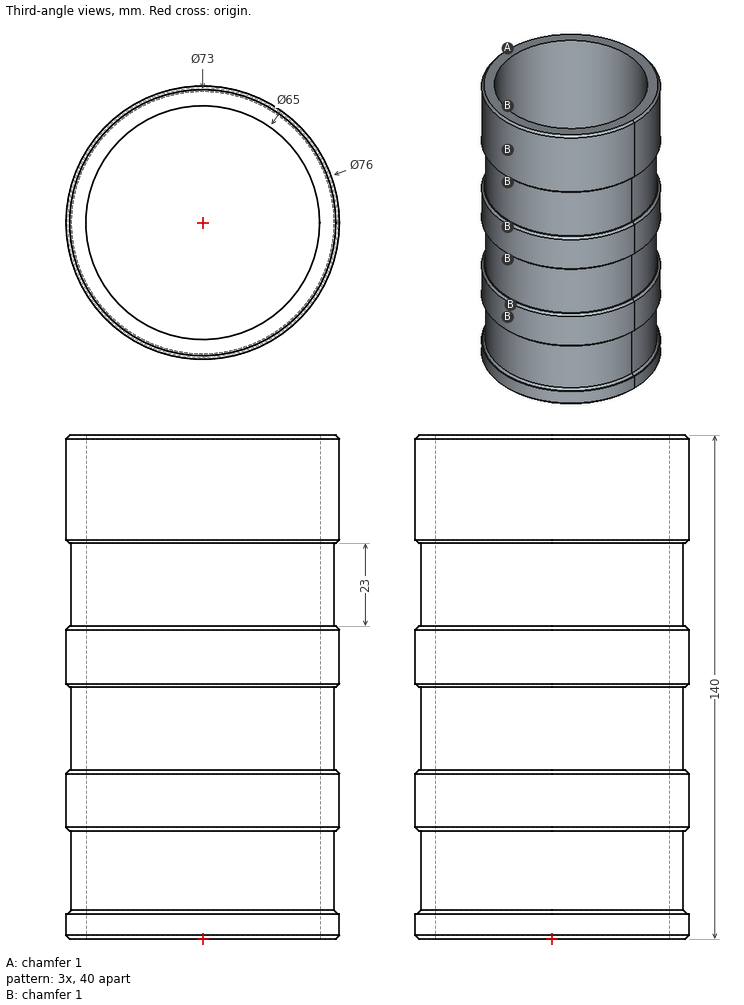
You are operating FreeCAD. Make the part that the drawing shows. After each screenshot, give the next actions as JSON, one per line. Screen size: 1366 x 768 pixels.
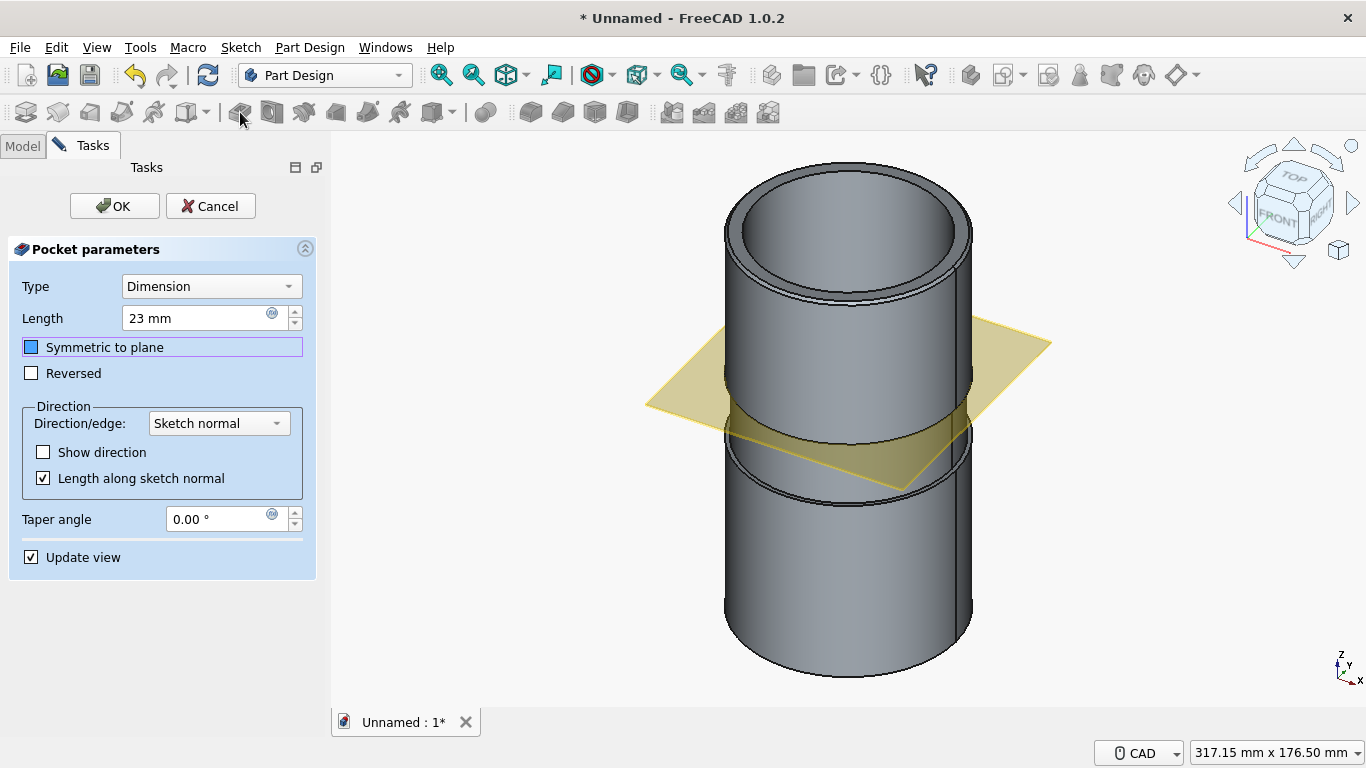
{"action": "left_click", "coordinate": [30, 373]}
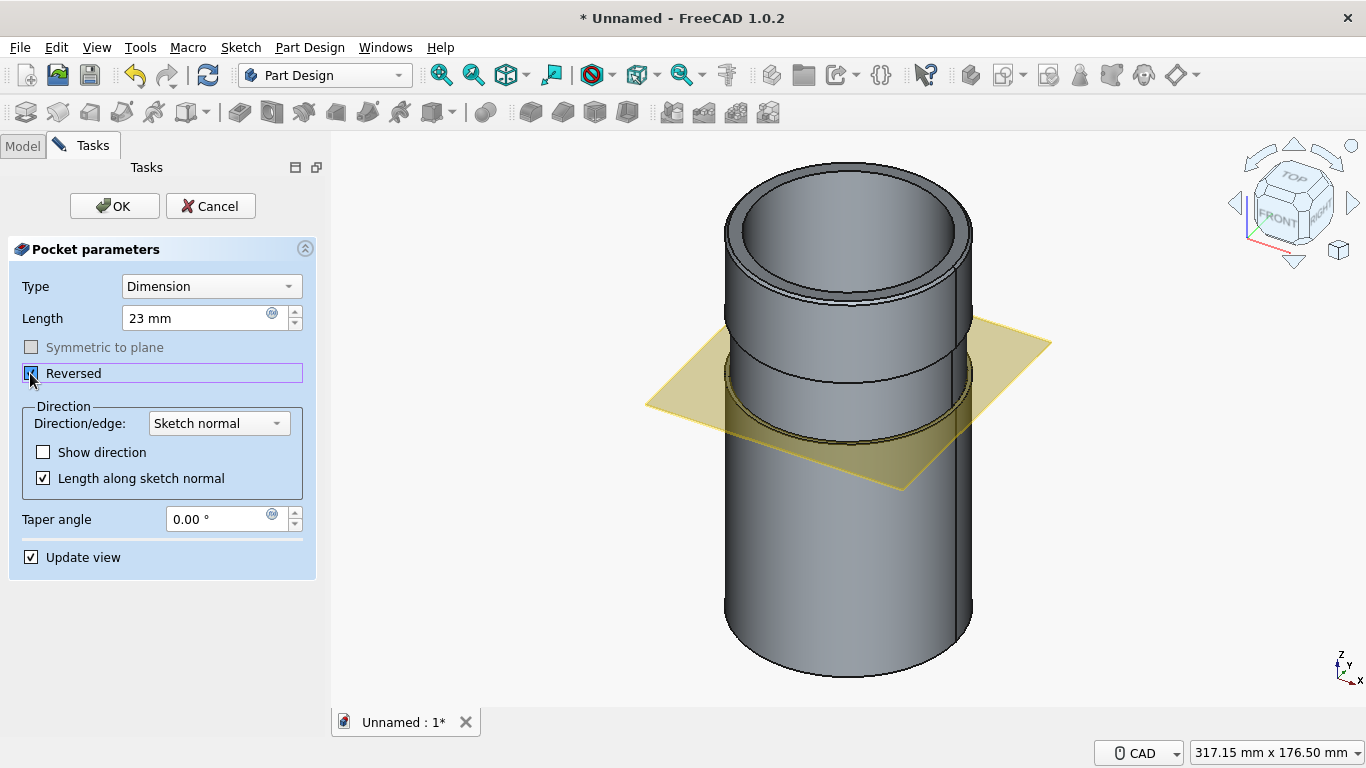
{"action": "left_click", "coordinate": [115, 206]}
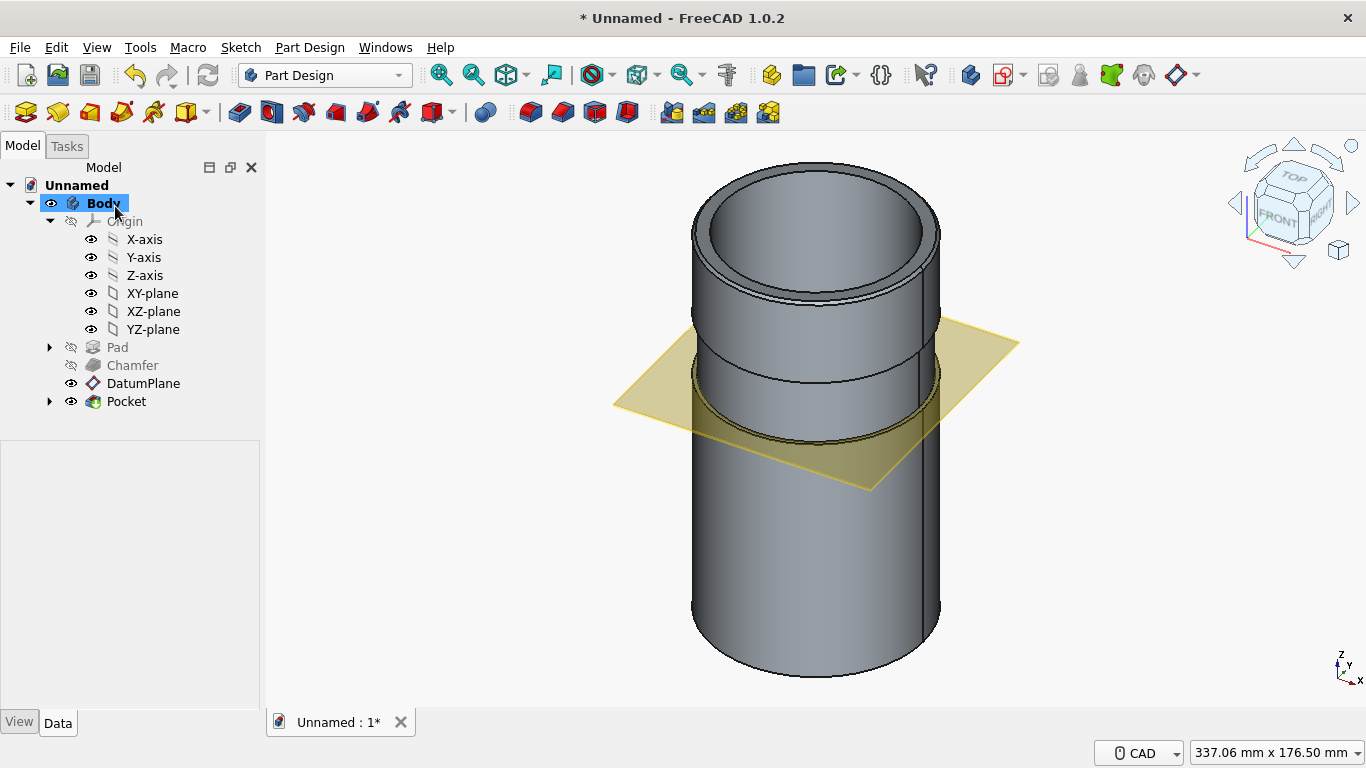
{"action": "left_click", "coordinate": [116, 383]}
{"action": "key", "text": "space"}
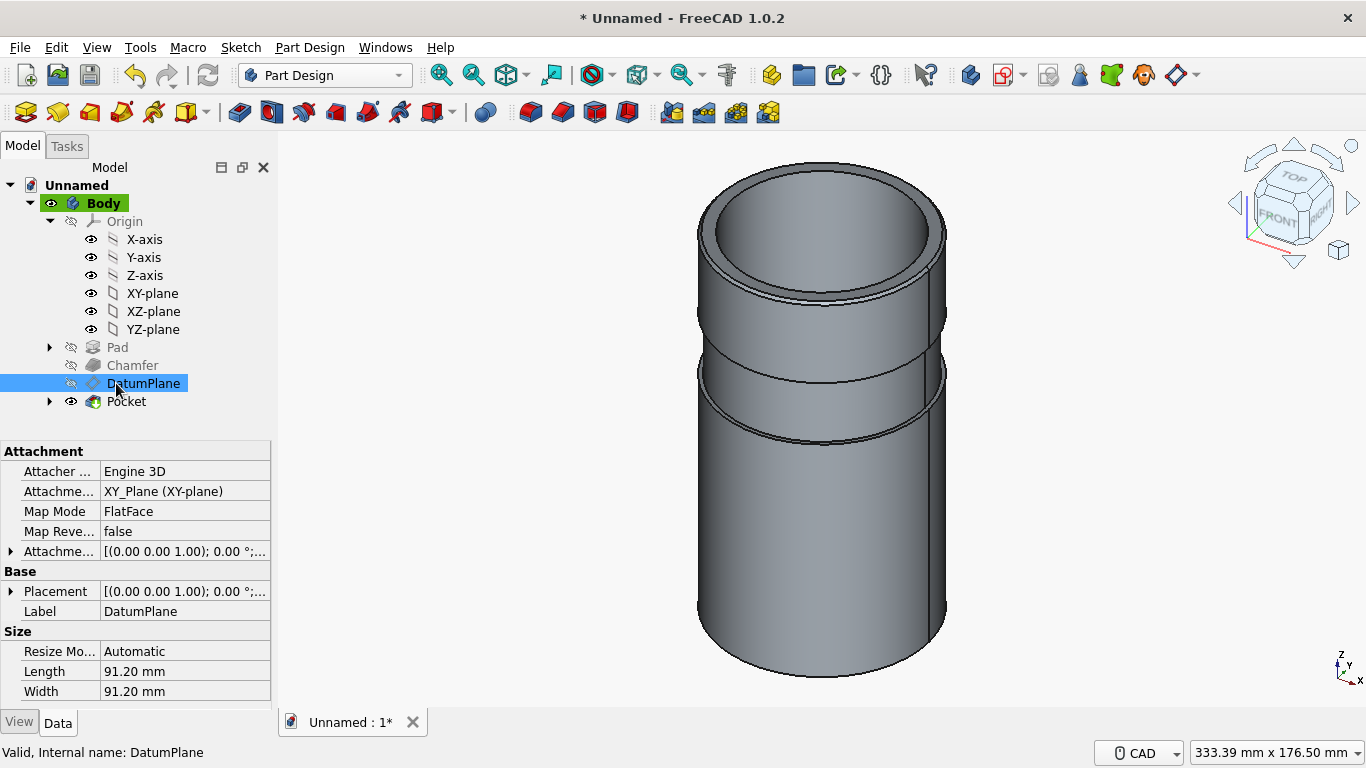
{"action": "left_click", "coordinate": [116, 401]}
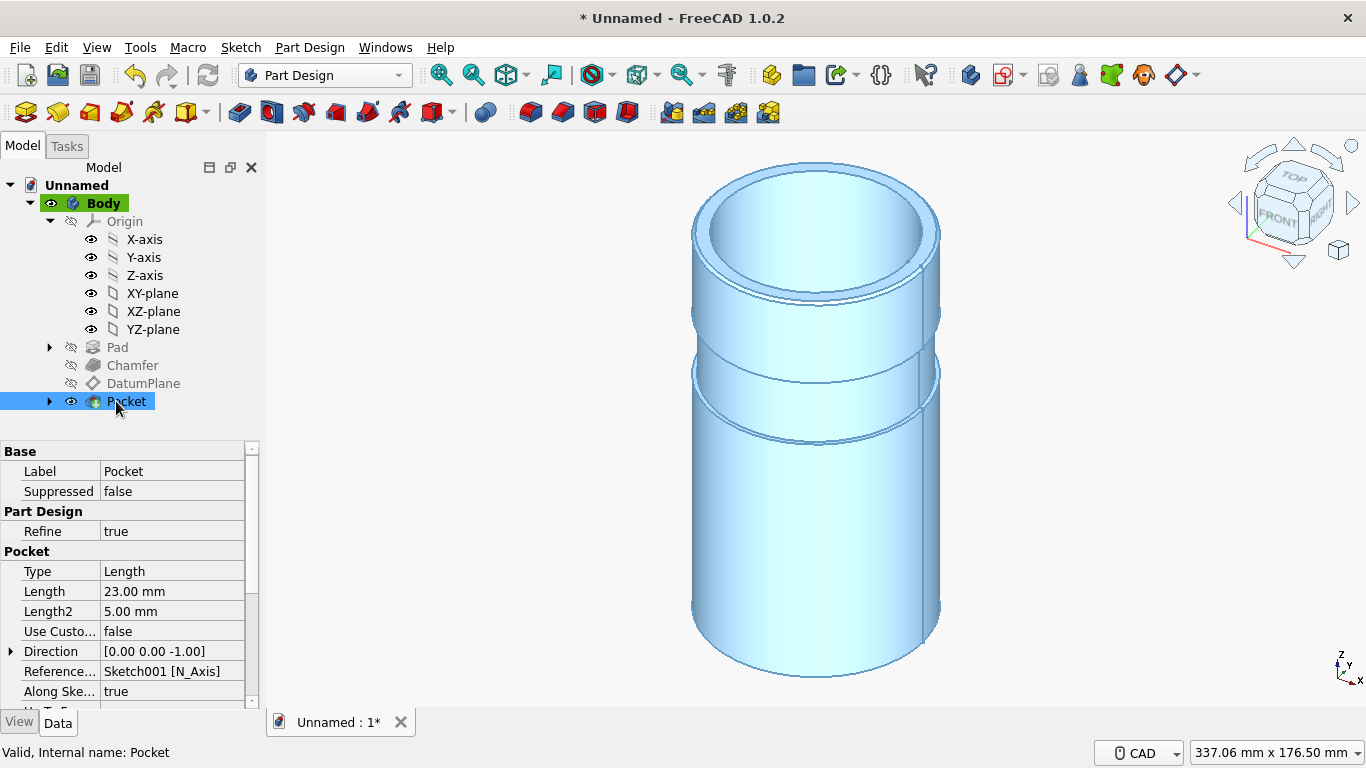
{"action": "left_click", "coordinate": [704, 112]}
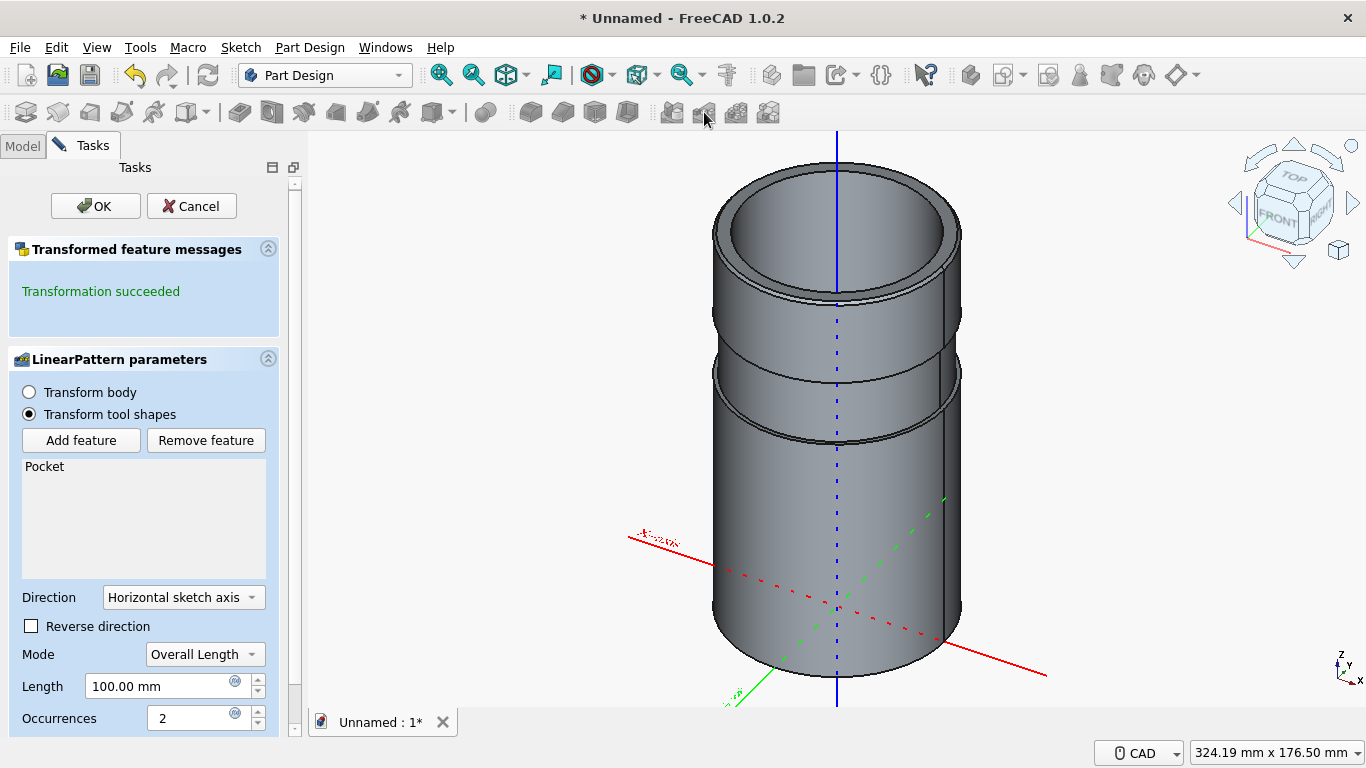
{"action": "left_click", "coordinate": [184, 598]}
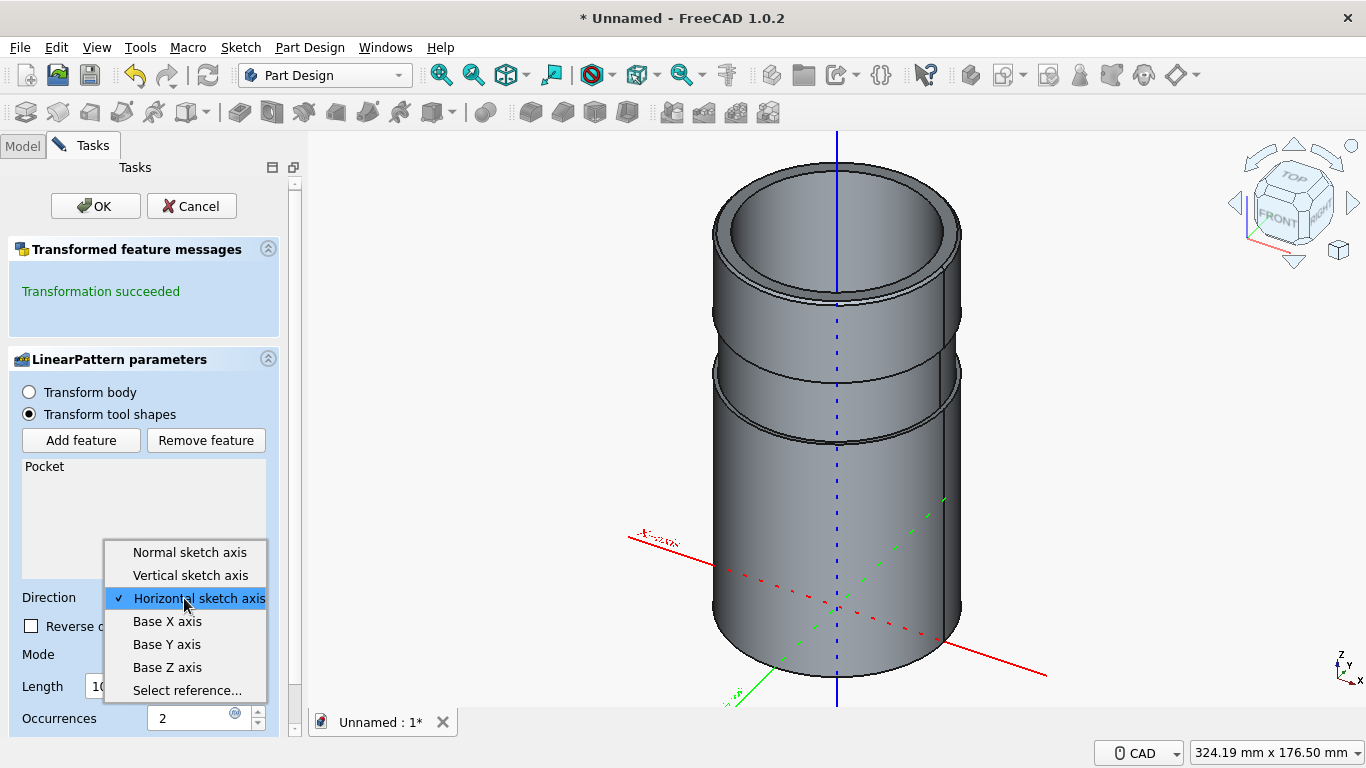
{"action": "left_click", "coordinate": [184, 668]}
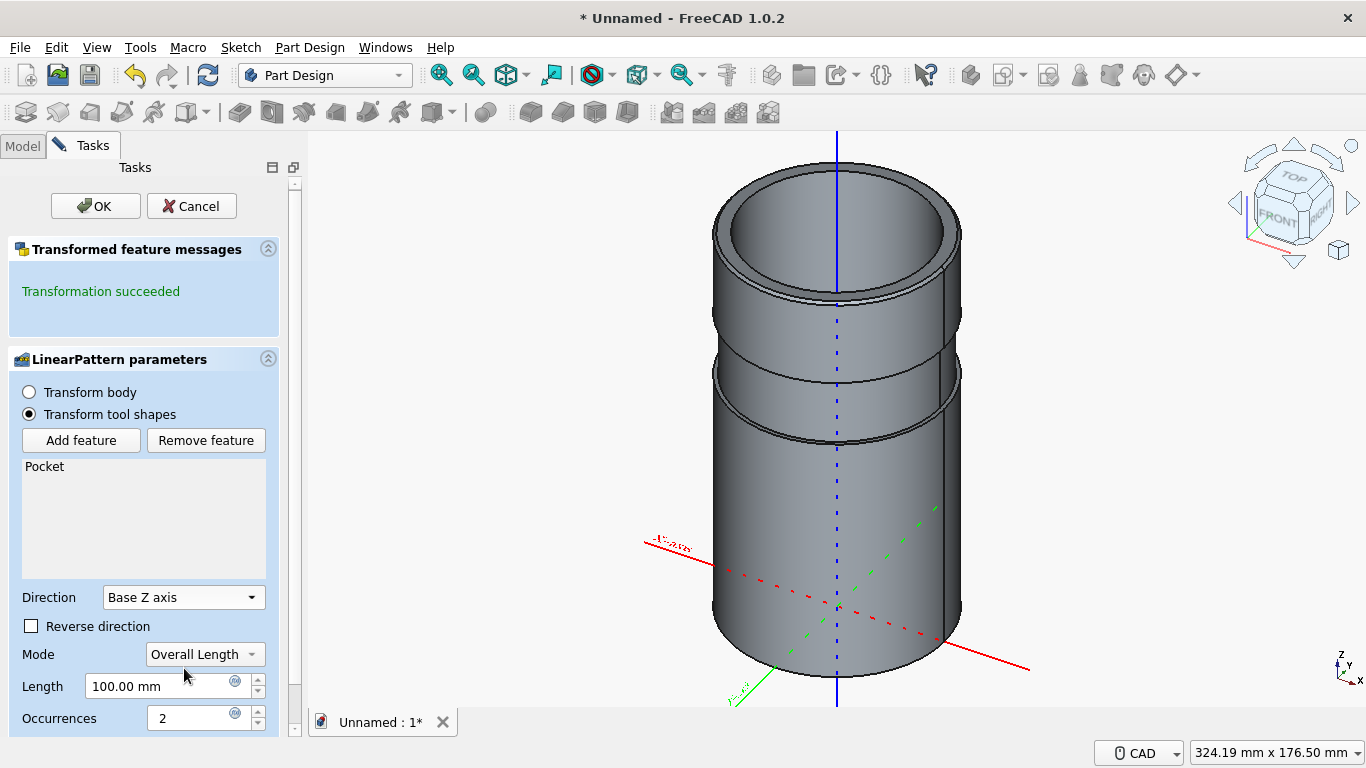
{"action": "left_click", "coordinate": [206, 654]}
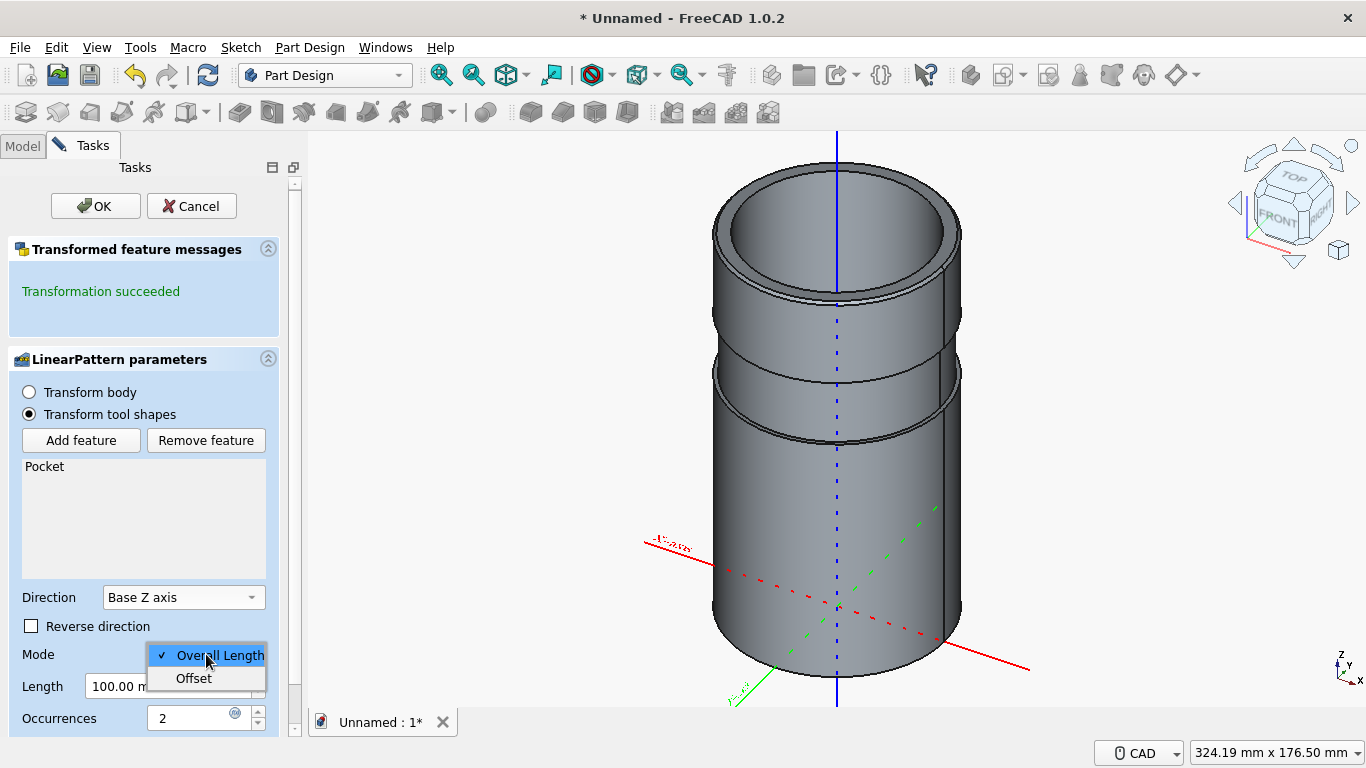
{"action": "left_click", "coordinate": [206, 678]}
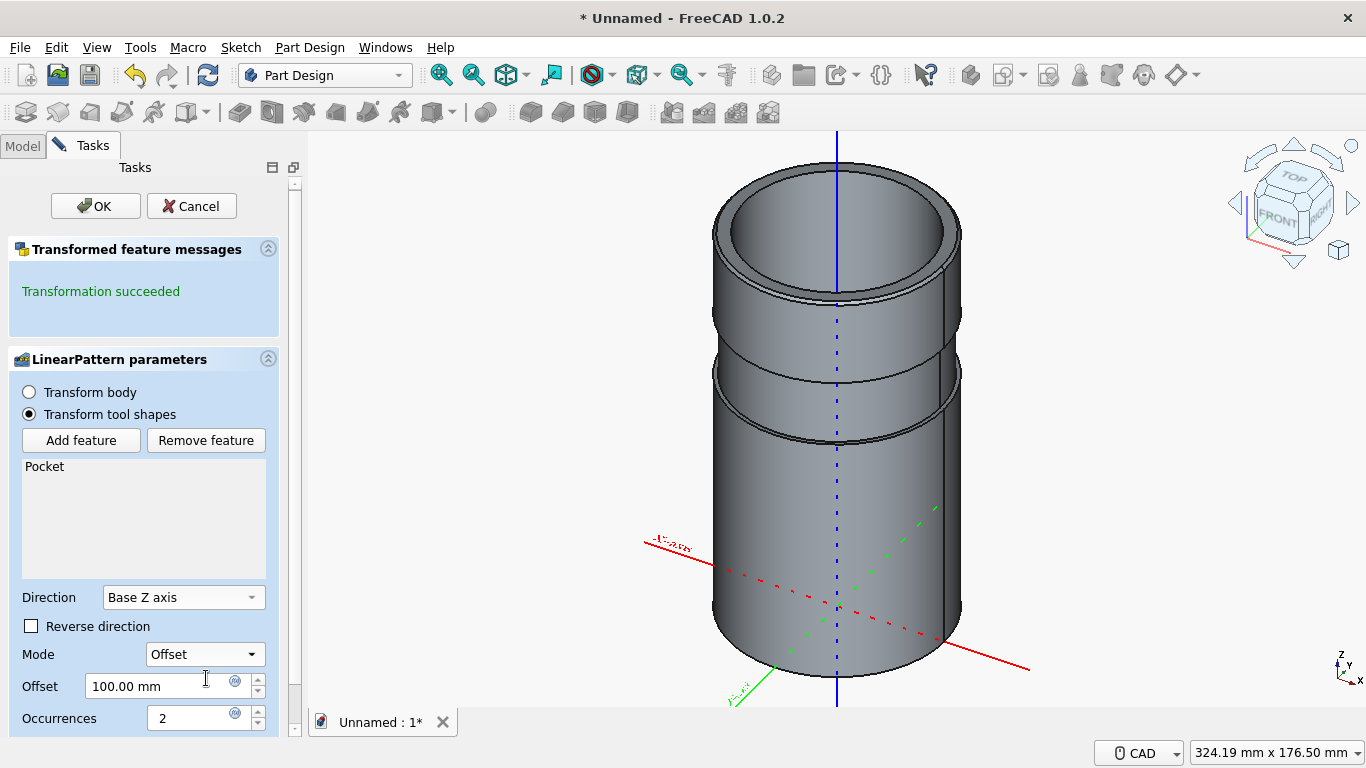
{"action": "triple_click", "coordinate": [168, 686]}